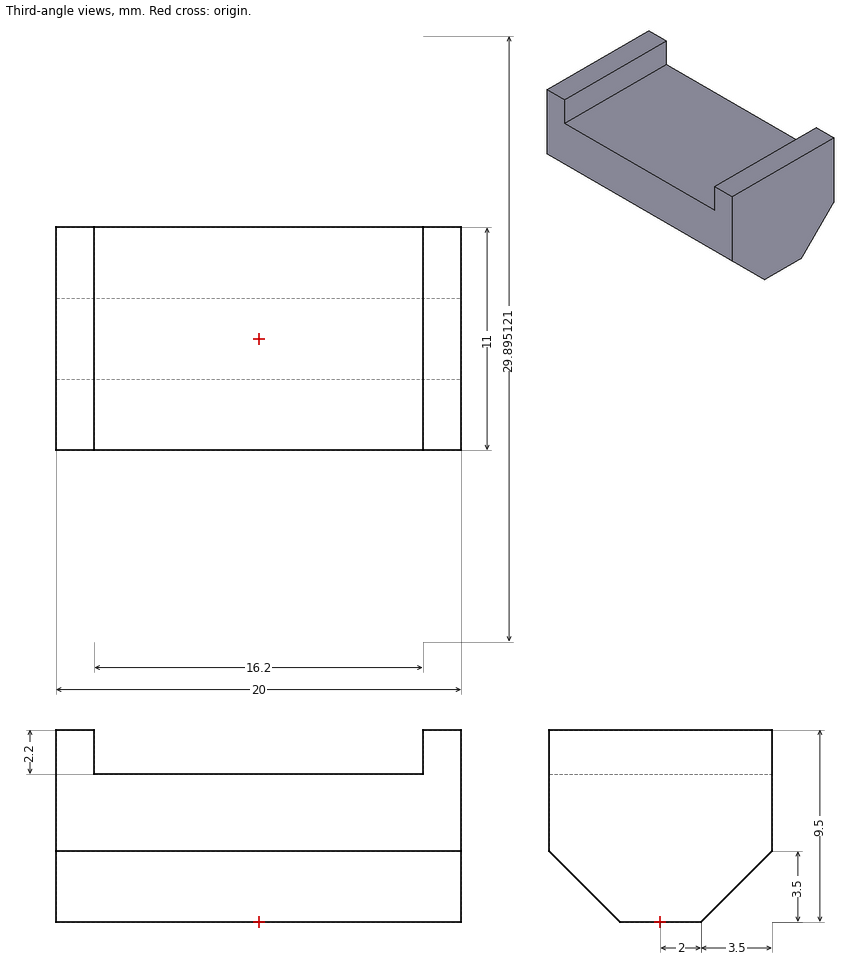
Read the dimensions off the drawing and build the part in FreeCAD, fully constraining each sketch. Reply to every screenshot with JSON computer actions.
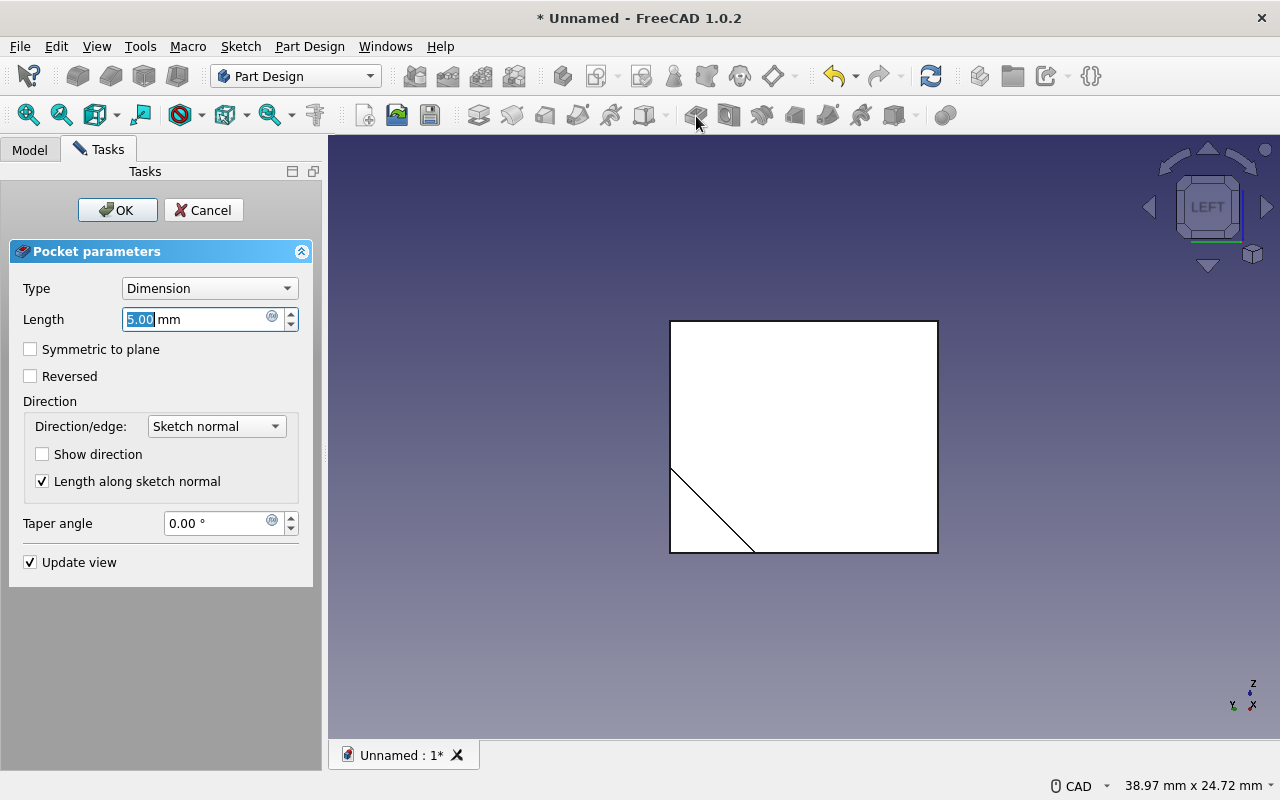
{"action": "left_click", "coordinate": [210, 288]}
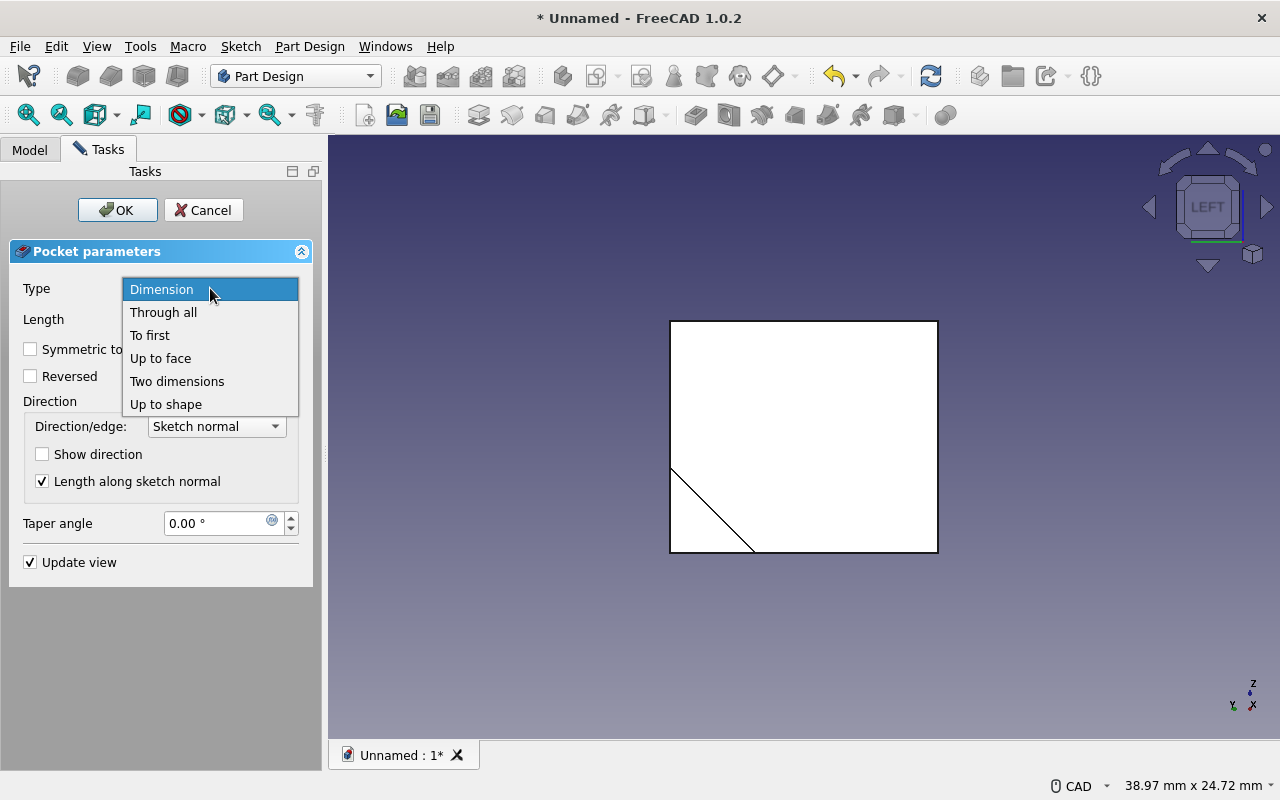
{"action": "left_click", "coordinate": [208, 312]}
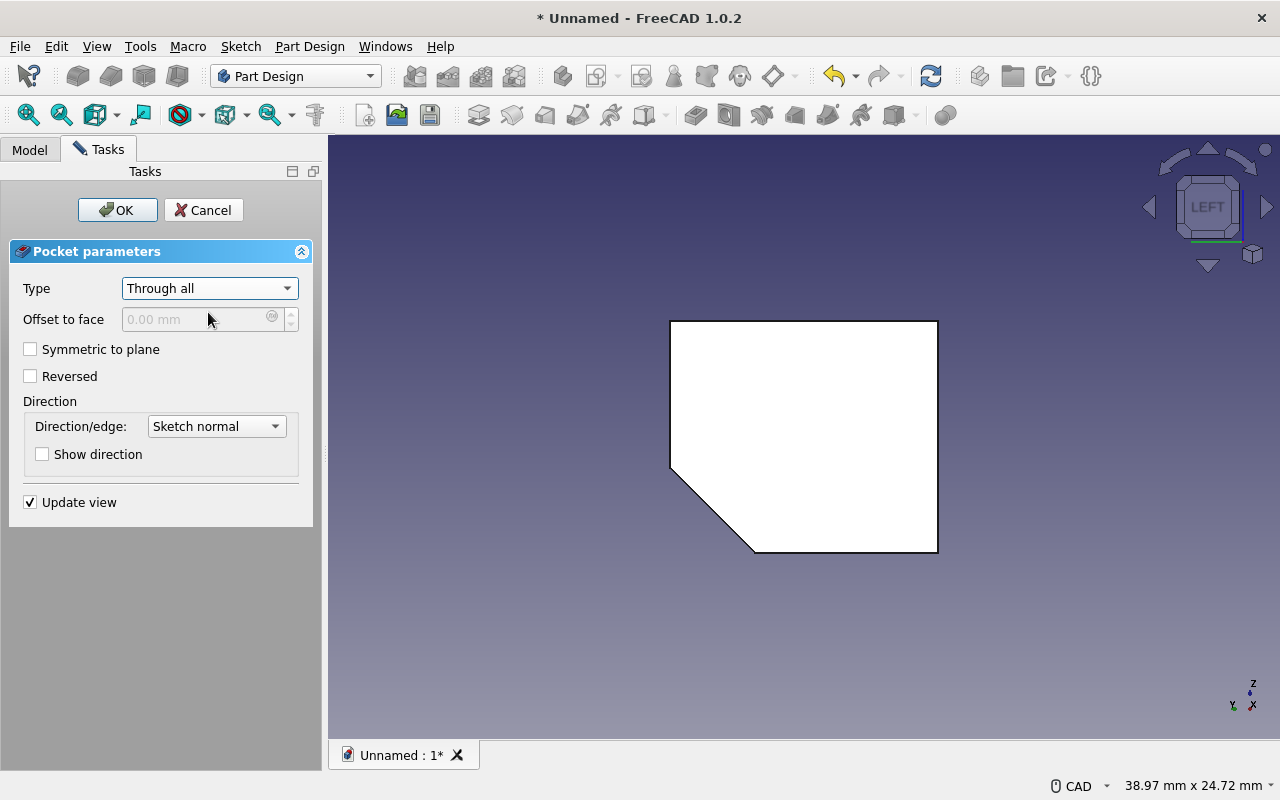
{"action": "left_click", "coordinate": [118, 210]}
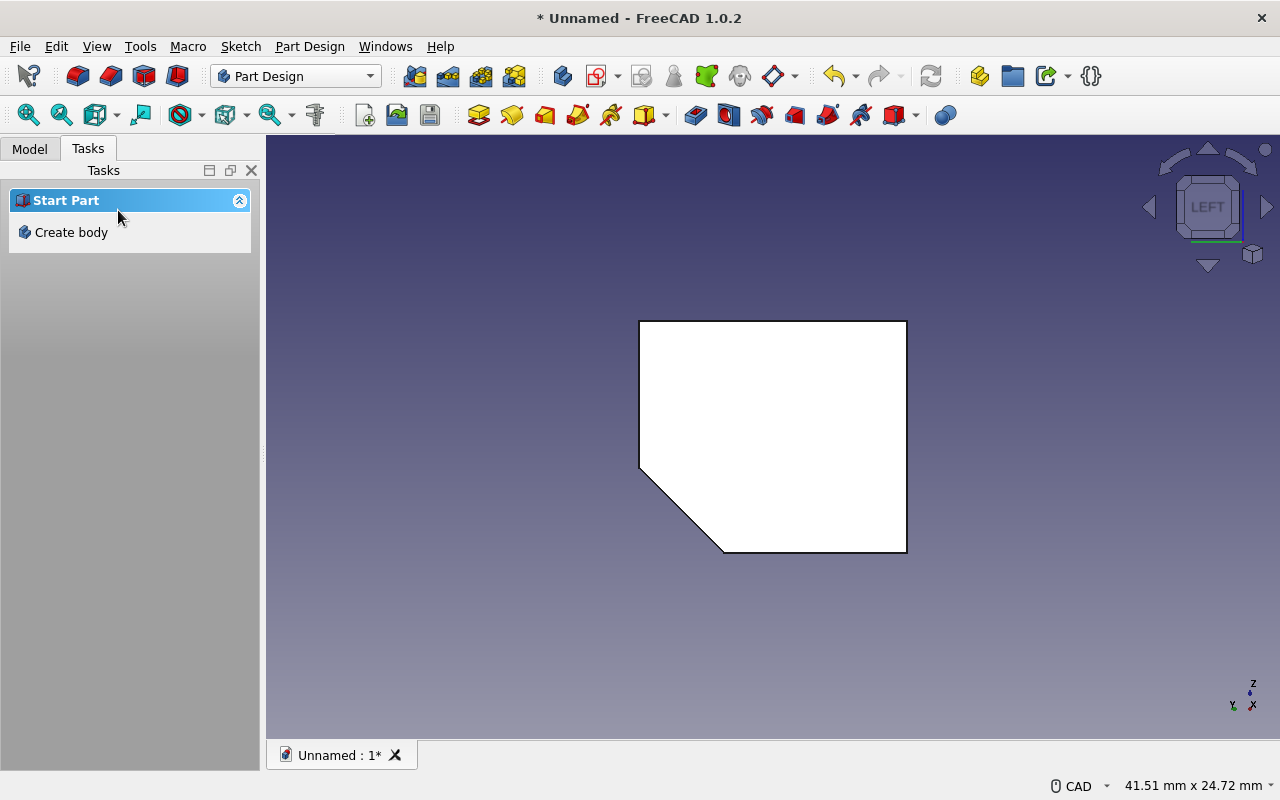
{"action": "left_click", "coordinate": [29, 116]}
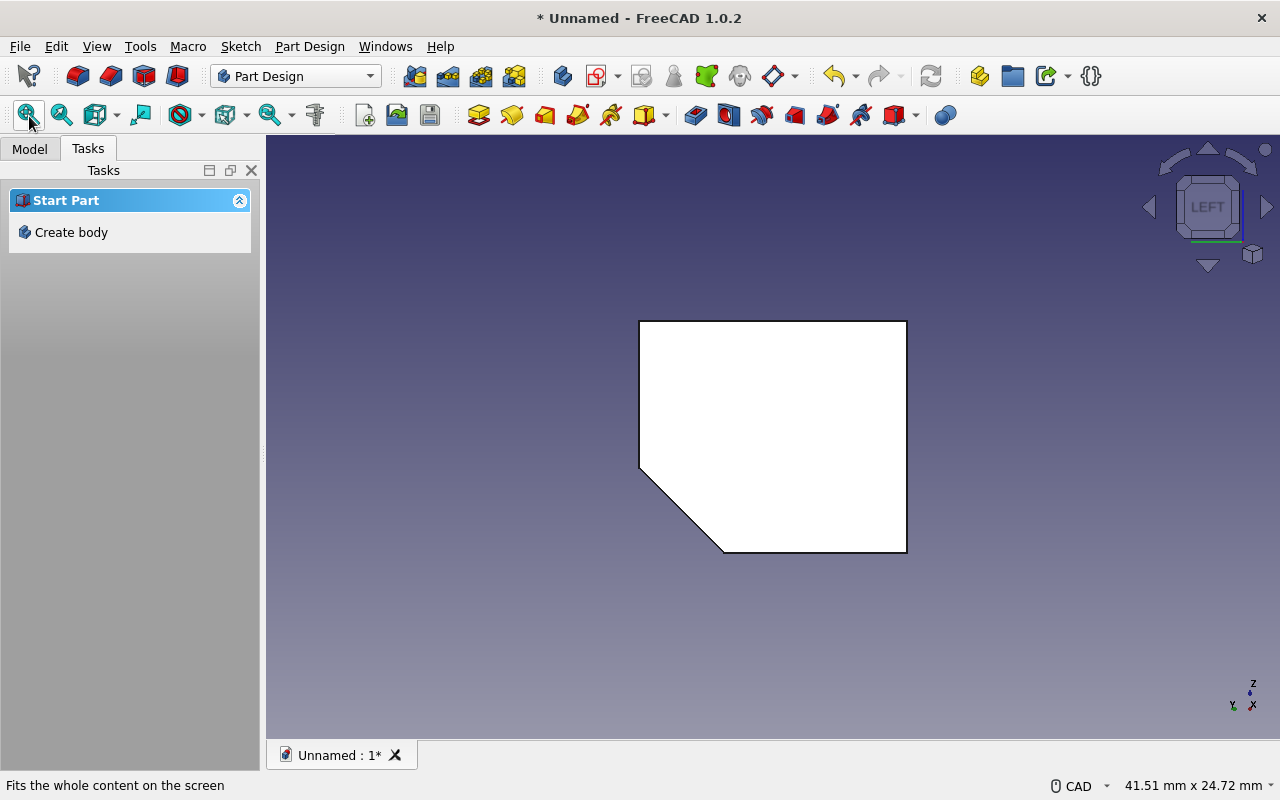
{"action": "left_click", "coordinate": [30, 148]}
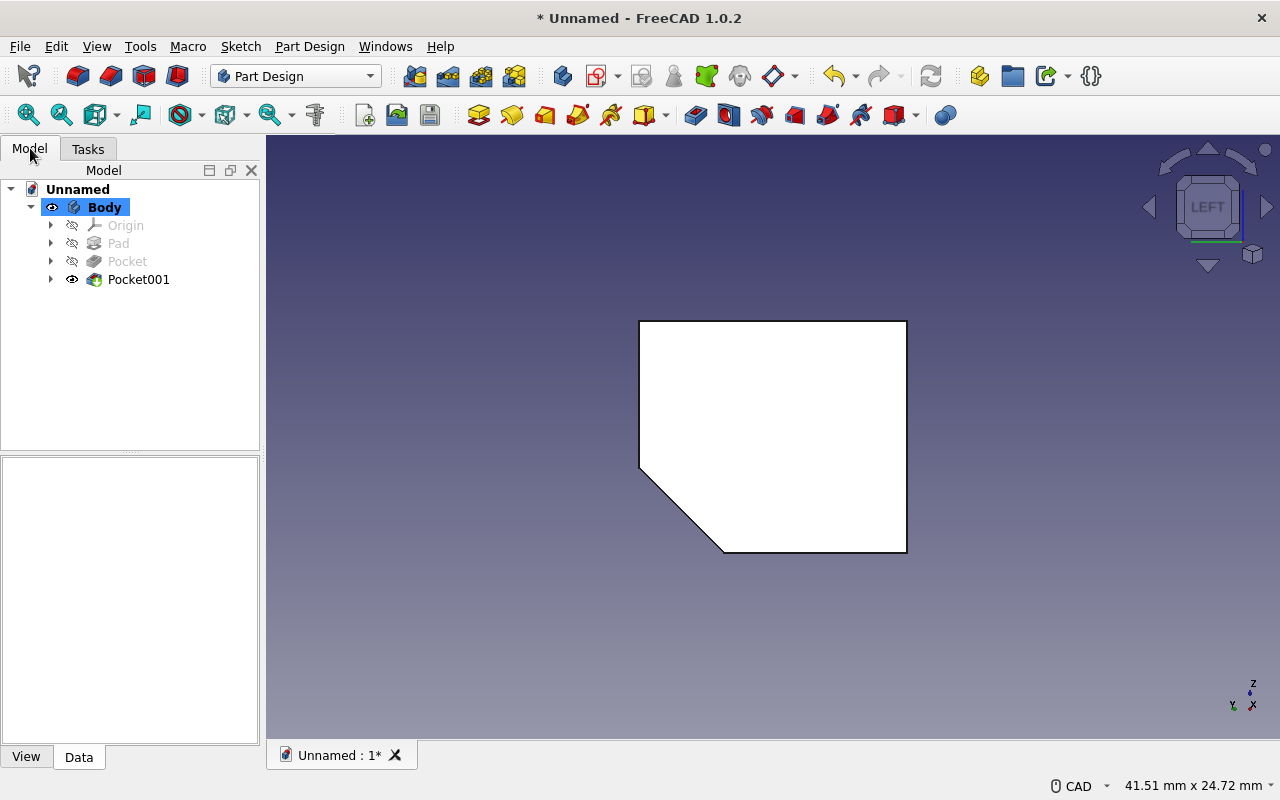
{"action": "left_click", "coordinate": [117, 279]}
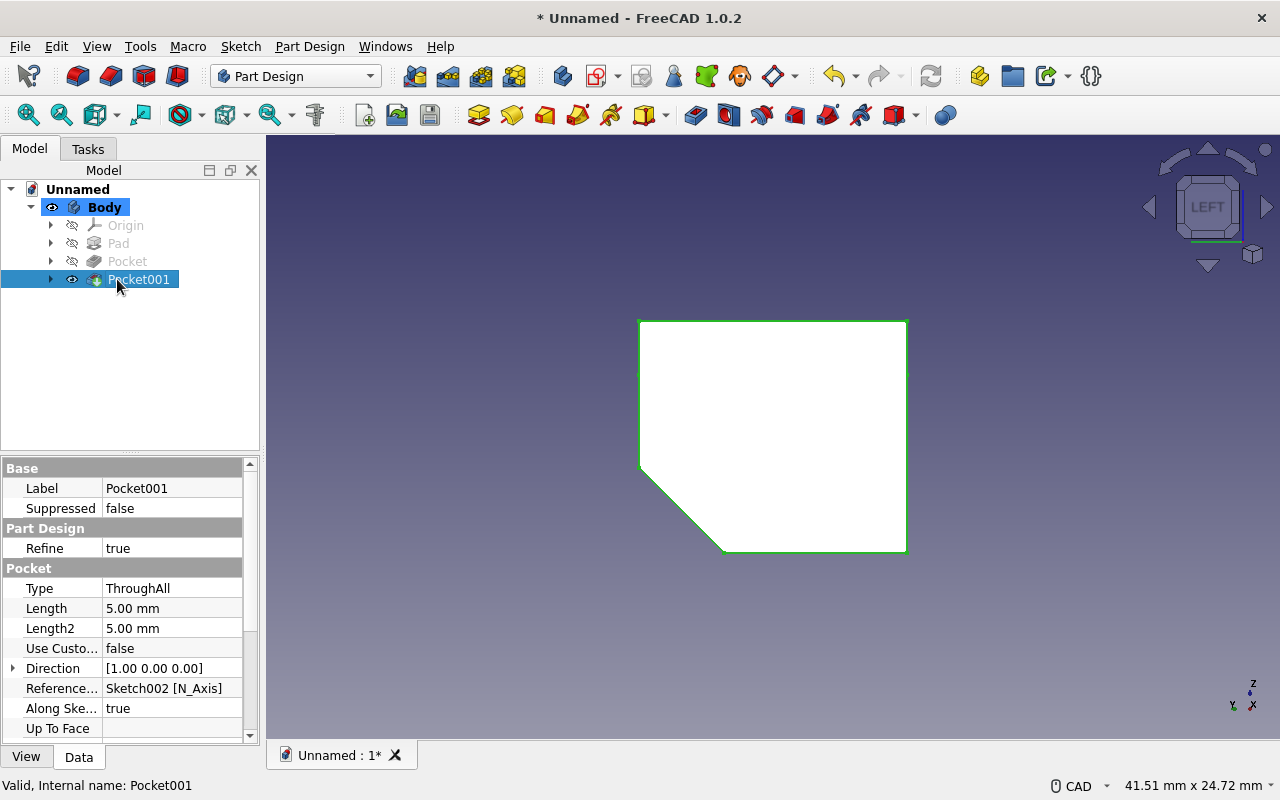
{"action": "left_click", "coordinate": [415, 76]}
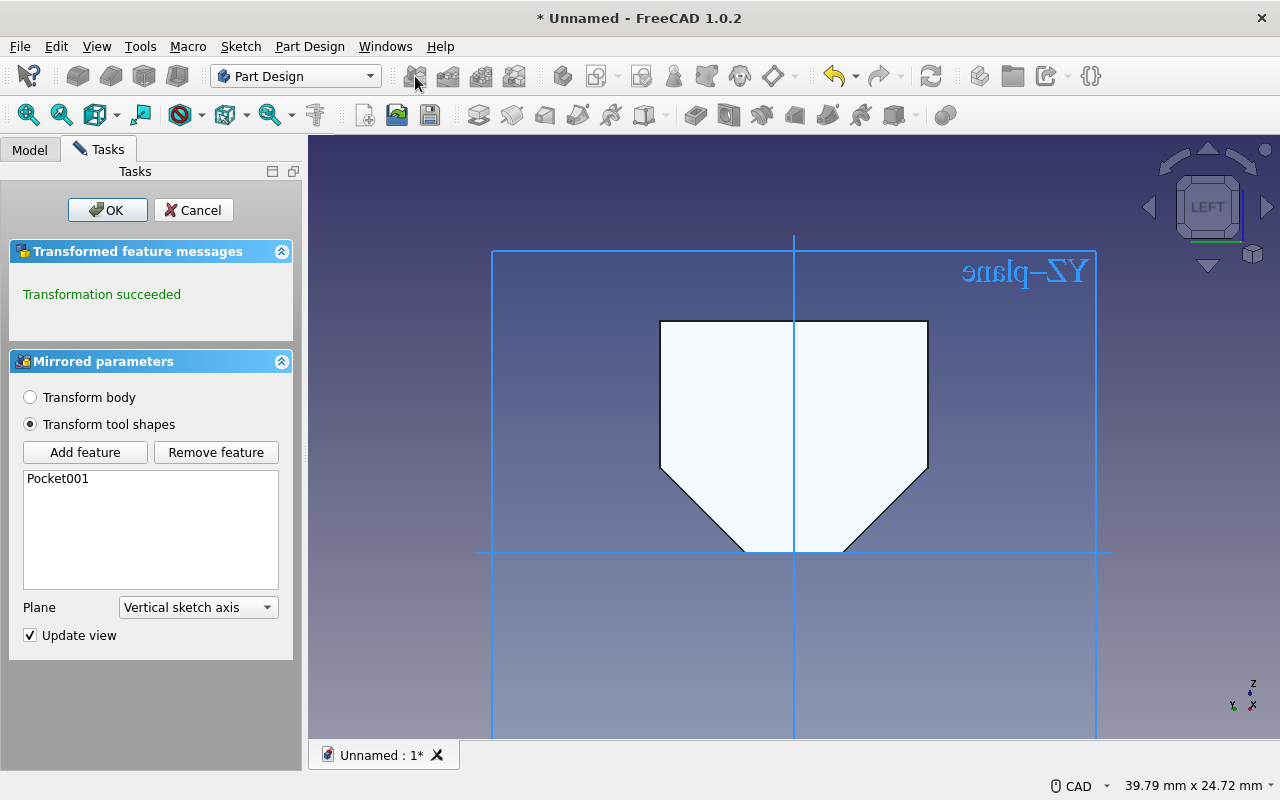
{"action": "left_click", "coordinate": [199, 608]}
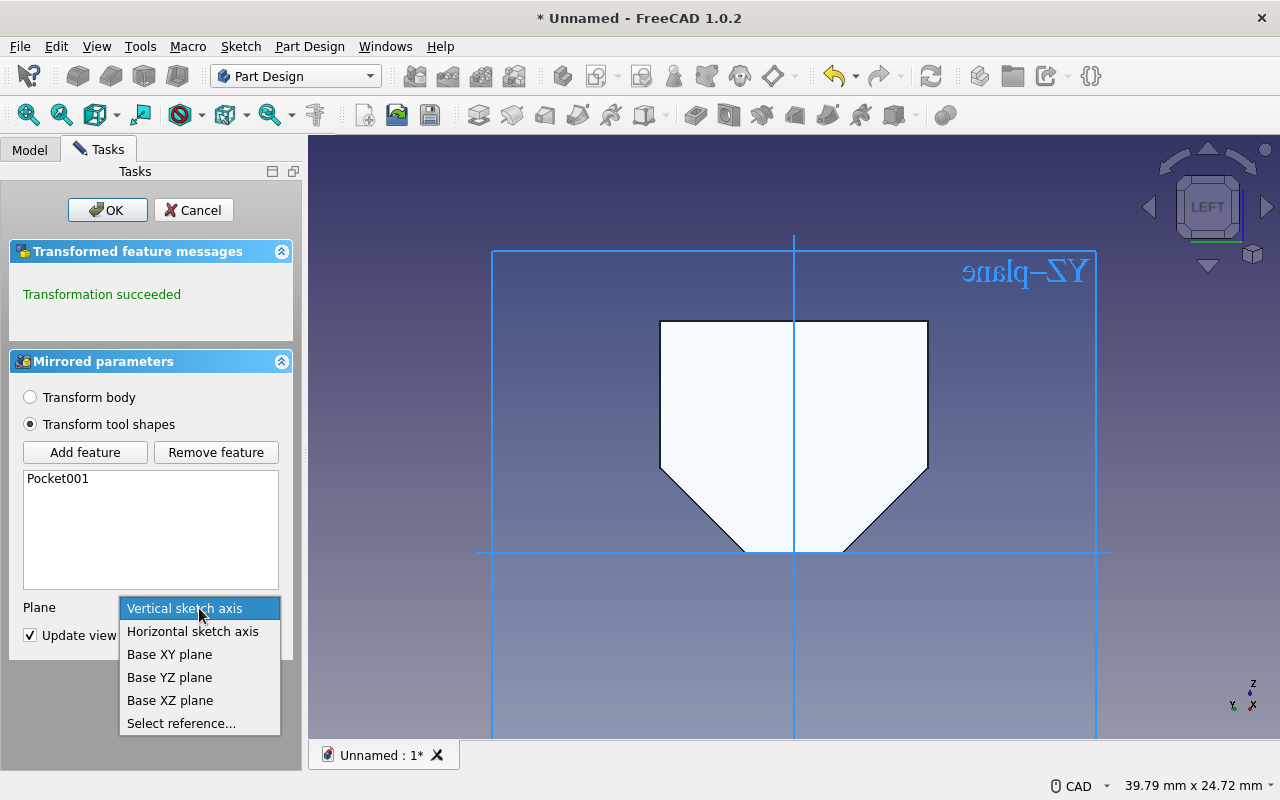
{"action": "left_click", "coordinate": [198, 700]}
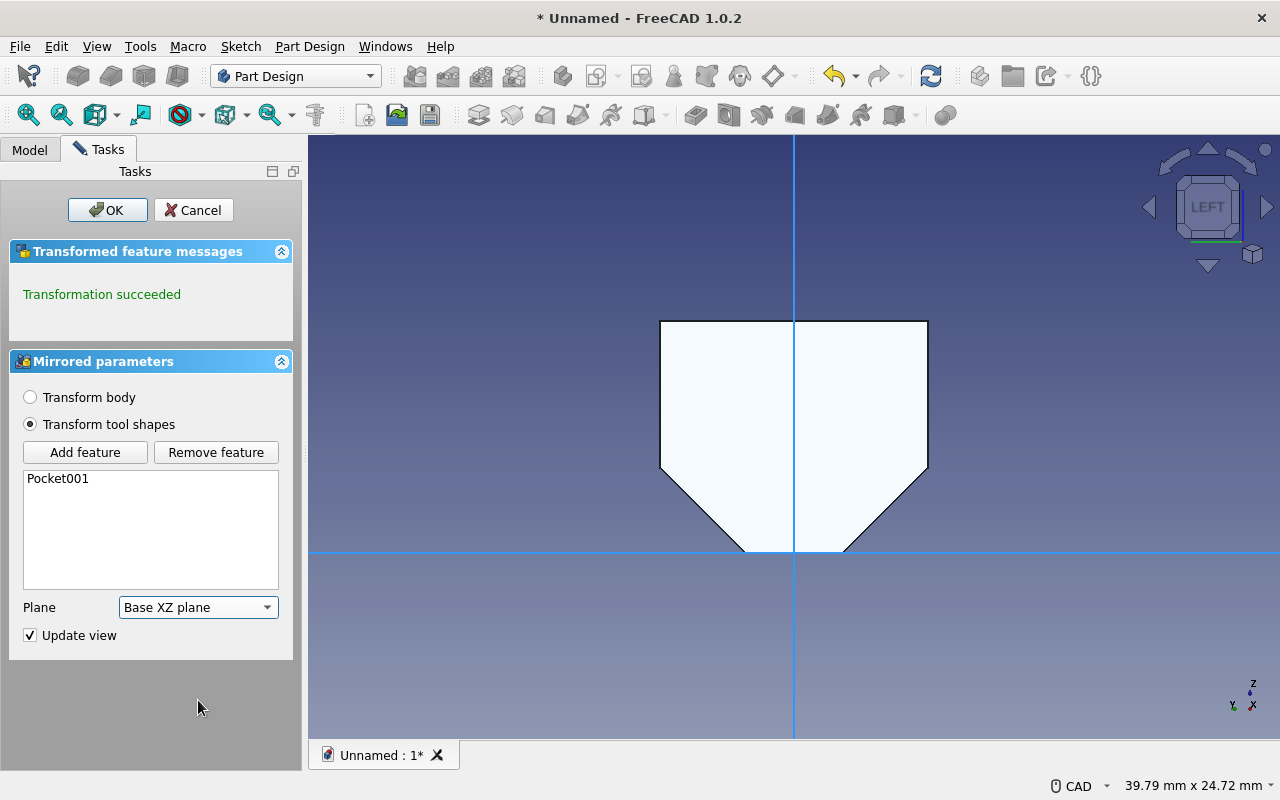
{"action": "left_click", "coordinate": [108, 210]}